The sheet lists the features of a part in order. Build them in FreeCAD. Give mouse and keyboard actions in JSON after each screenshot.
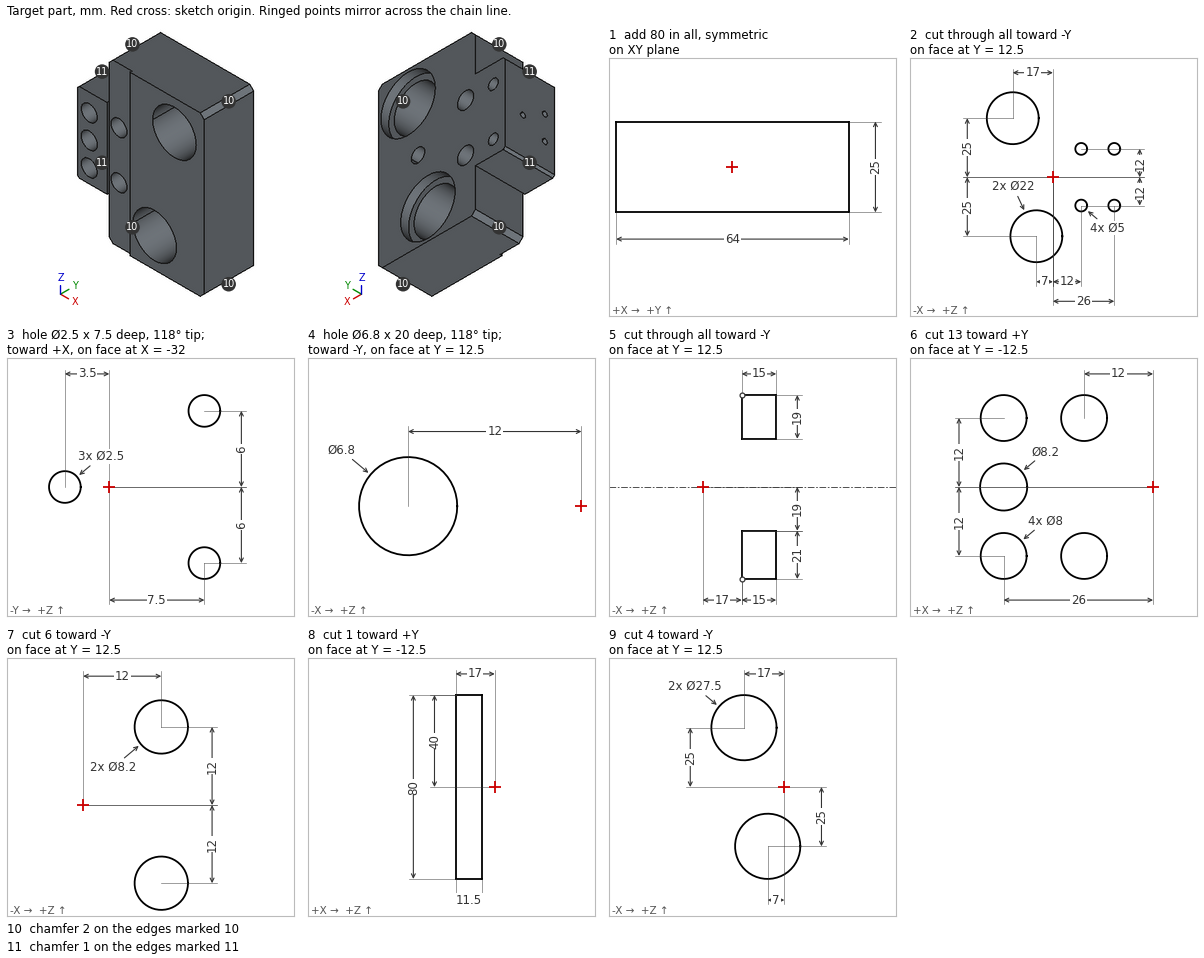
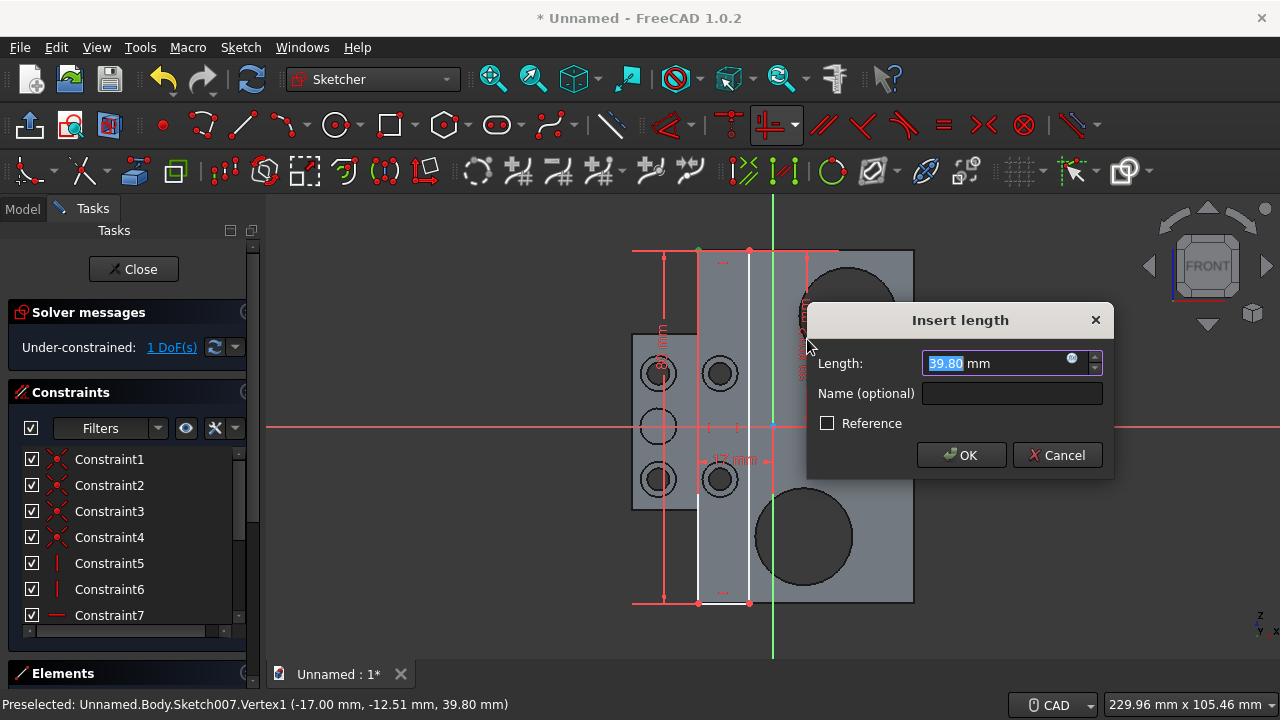
{"action": "type", "text": "40"}
{"action": "key", "text": "Return"}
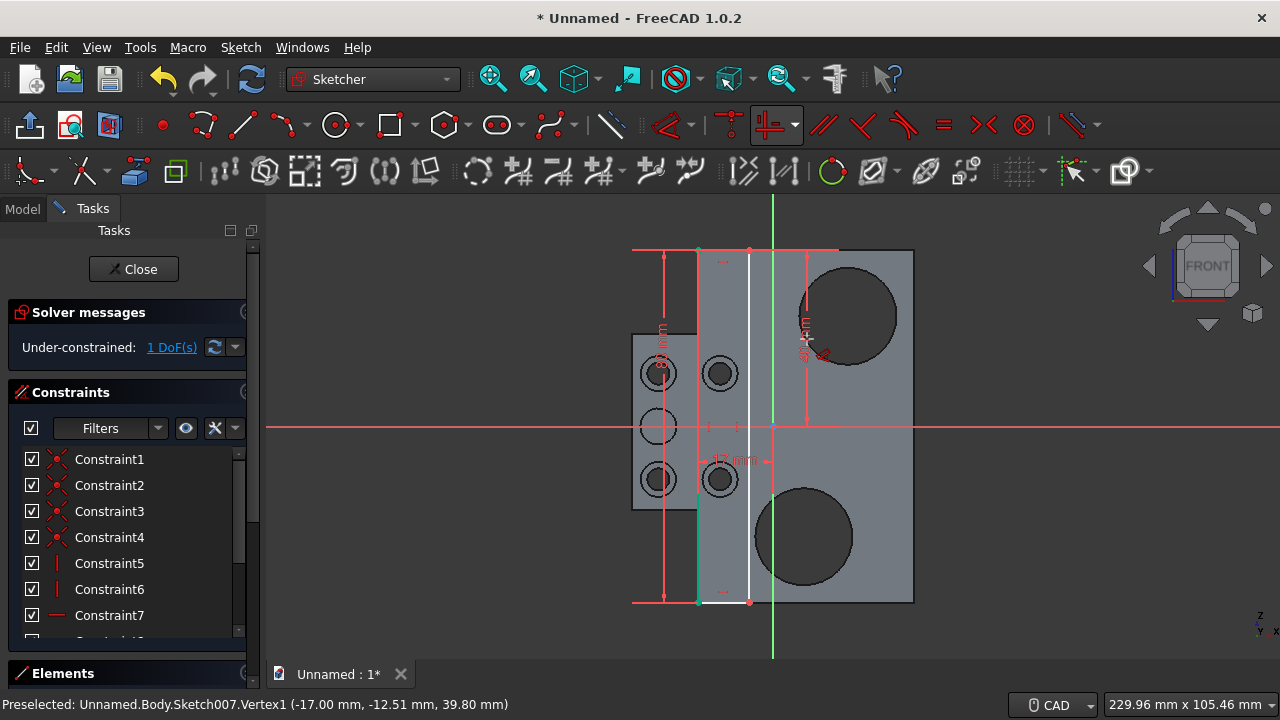
{"action": "left_click", "coordinate": [713, 603]}
{"action": "left_click", "coordinate": [724, 569]}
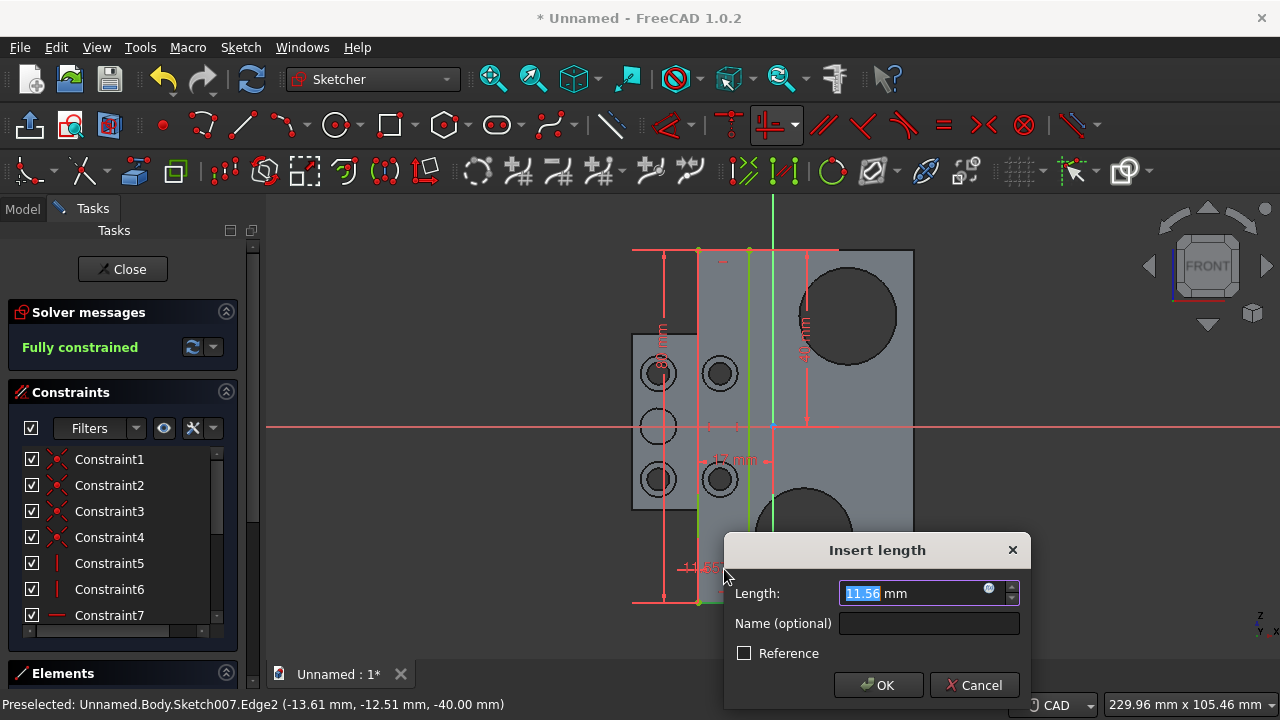
{"action": "type", "text": "11.5"}
{"action": "key", "text": "Return"}
{"action": "key", "text": "Escape"}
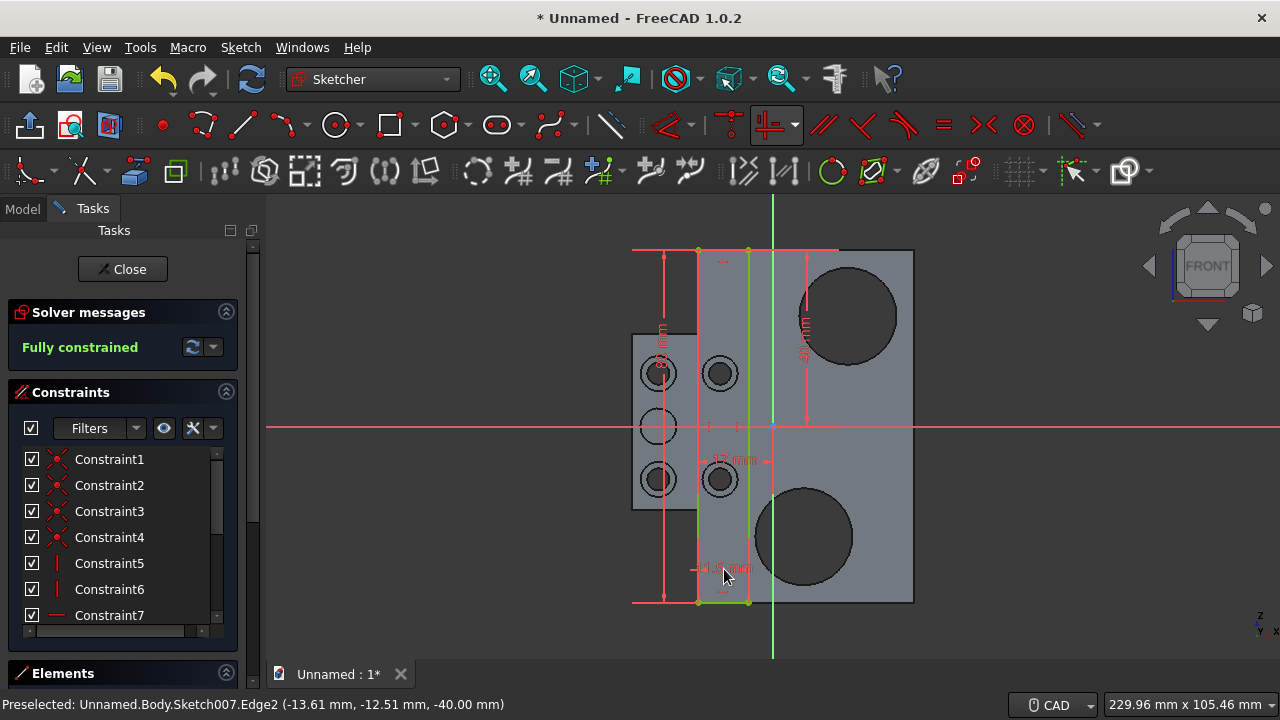
{"action": "left_click", "coordinate": [123, 269]}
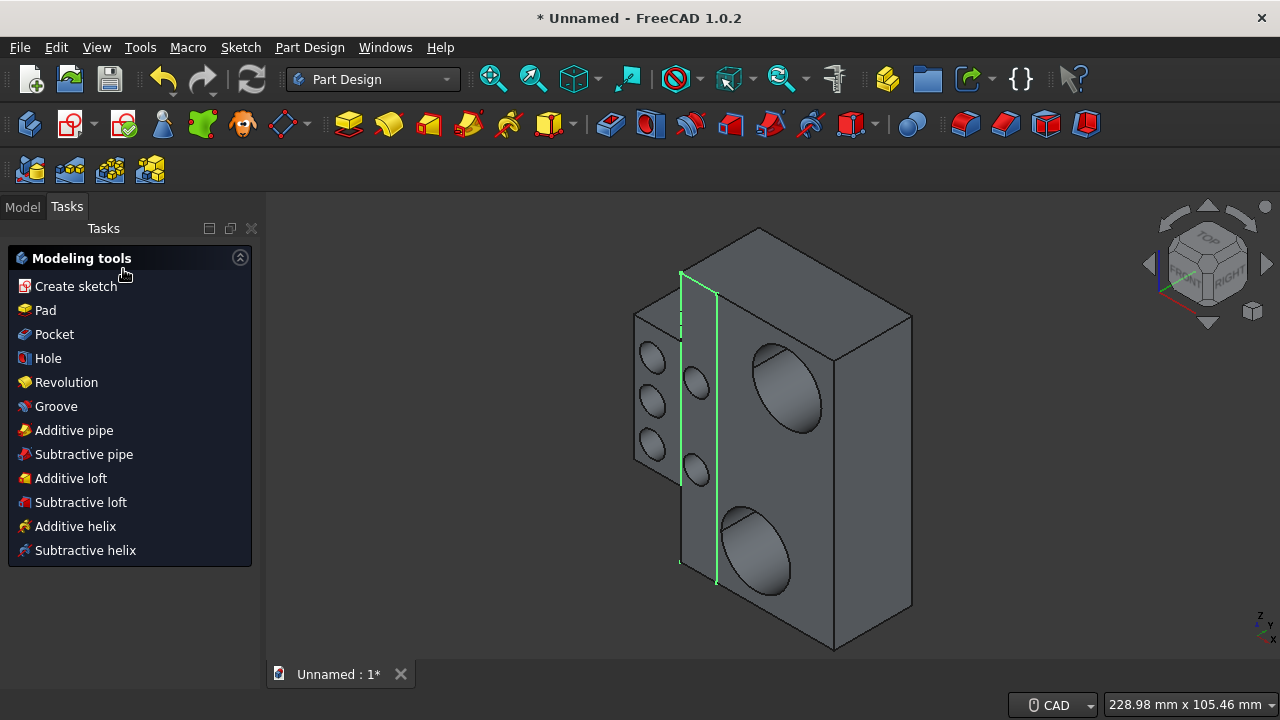
{"action": "left_click", "coordinate": [612, 124]}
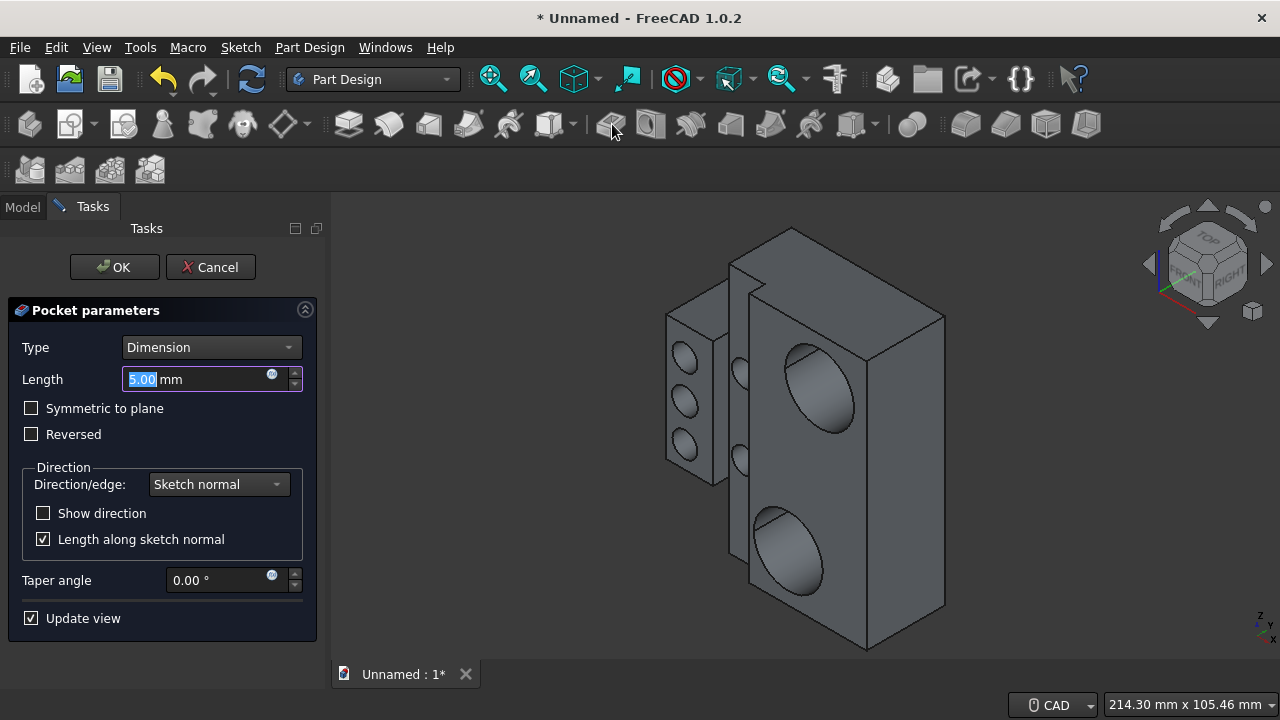
{"action": "type", "text": "1"}
{"action": "key", "text": "Tab"}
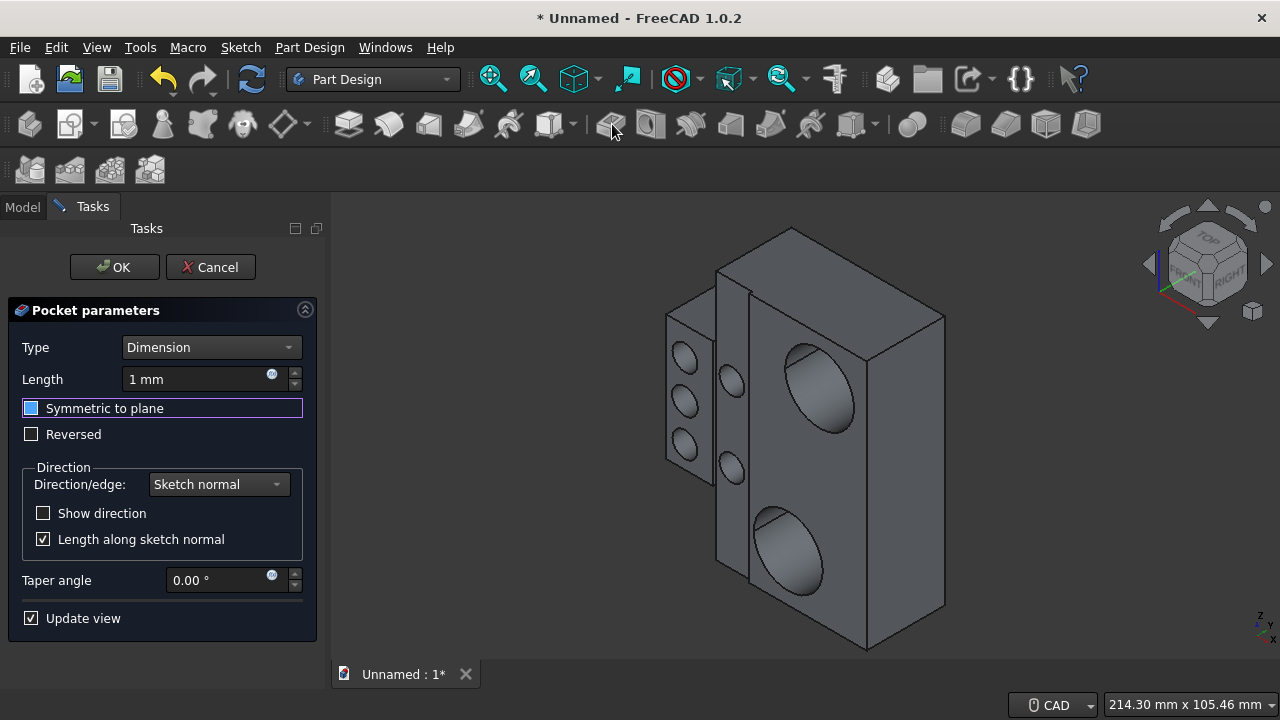
{"action": "left_click", "coordinate": [115, 267]}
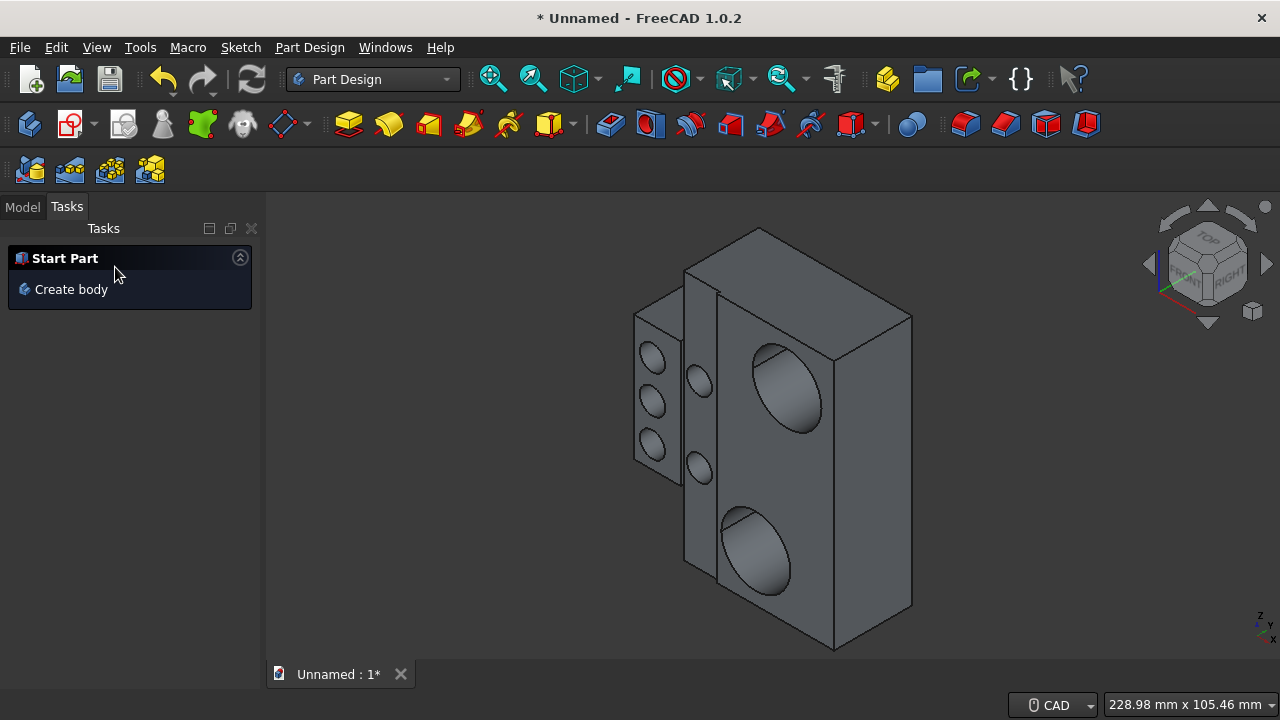
{"action": "key", "text": "4"}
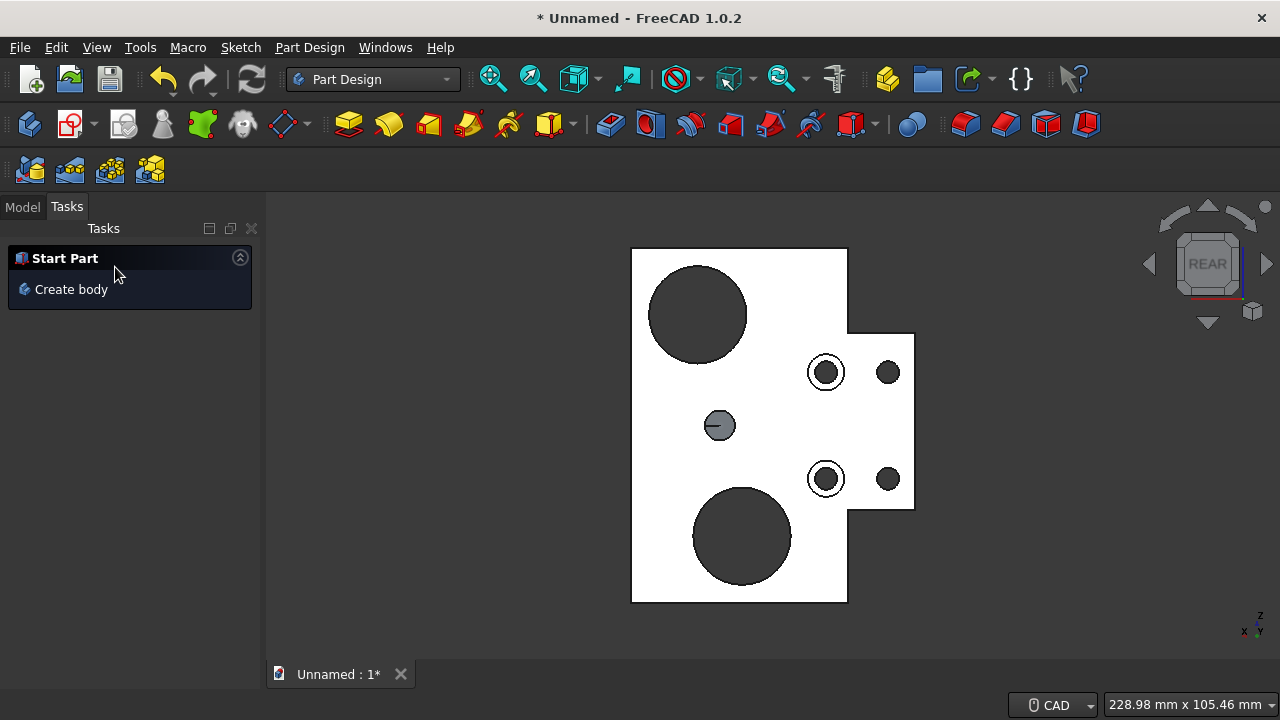
{"action": "left_click", "coordinate": [854, 425]}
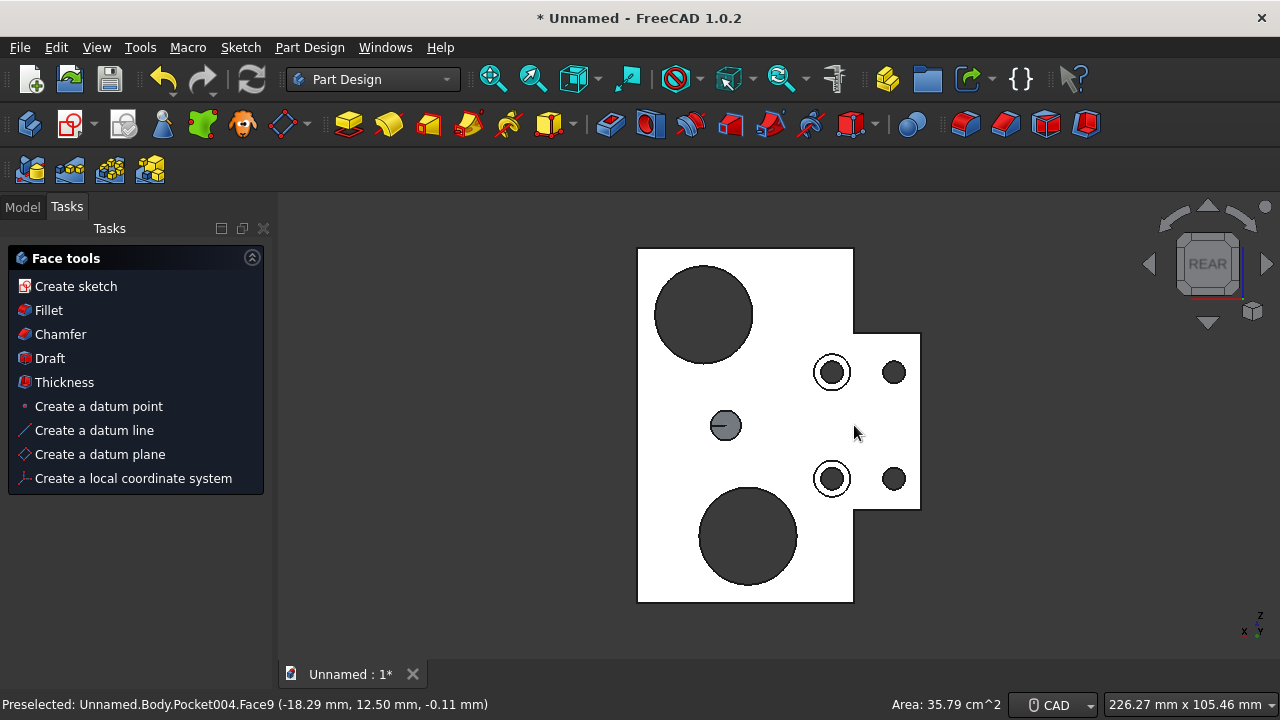
{"action": "left_click", "coordinate": [70, 124]}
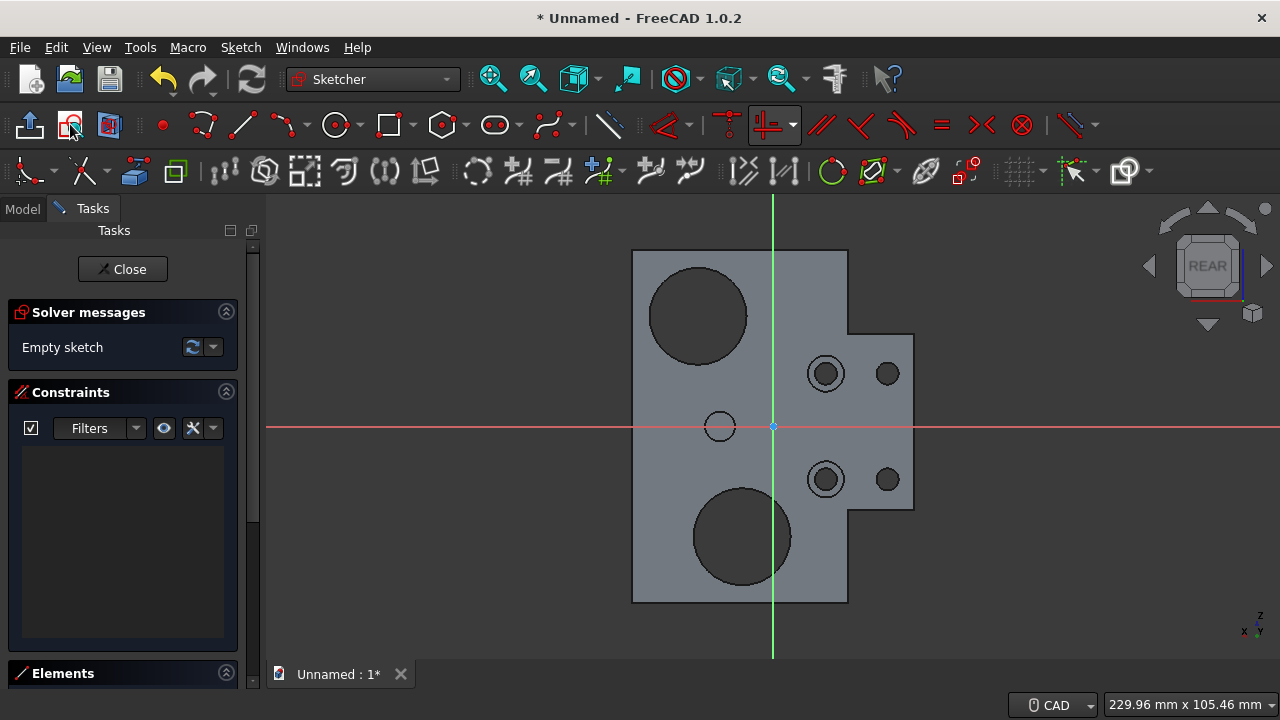
{"action": "left_click", "coordinate": [336, 126]}